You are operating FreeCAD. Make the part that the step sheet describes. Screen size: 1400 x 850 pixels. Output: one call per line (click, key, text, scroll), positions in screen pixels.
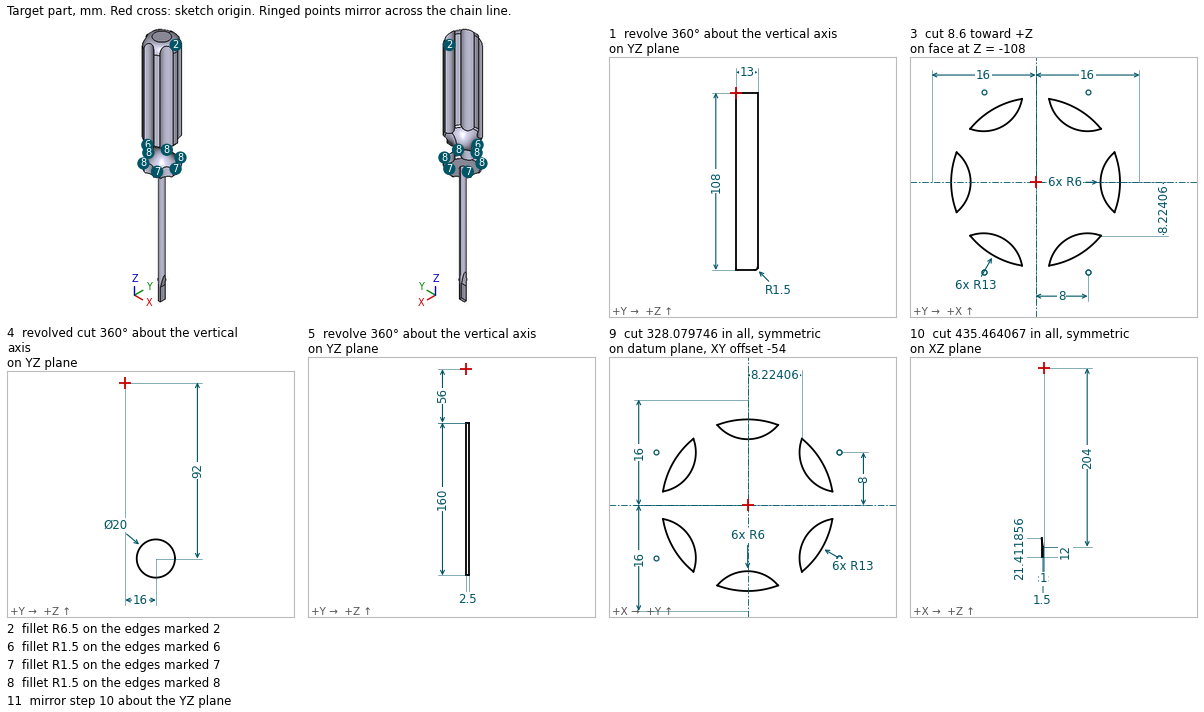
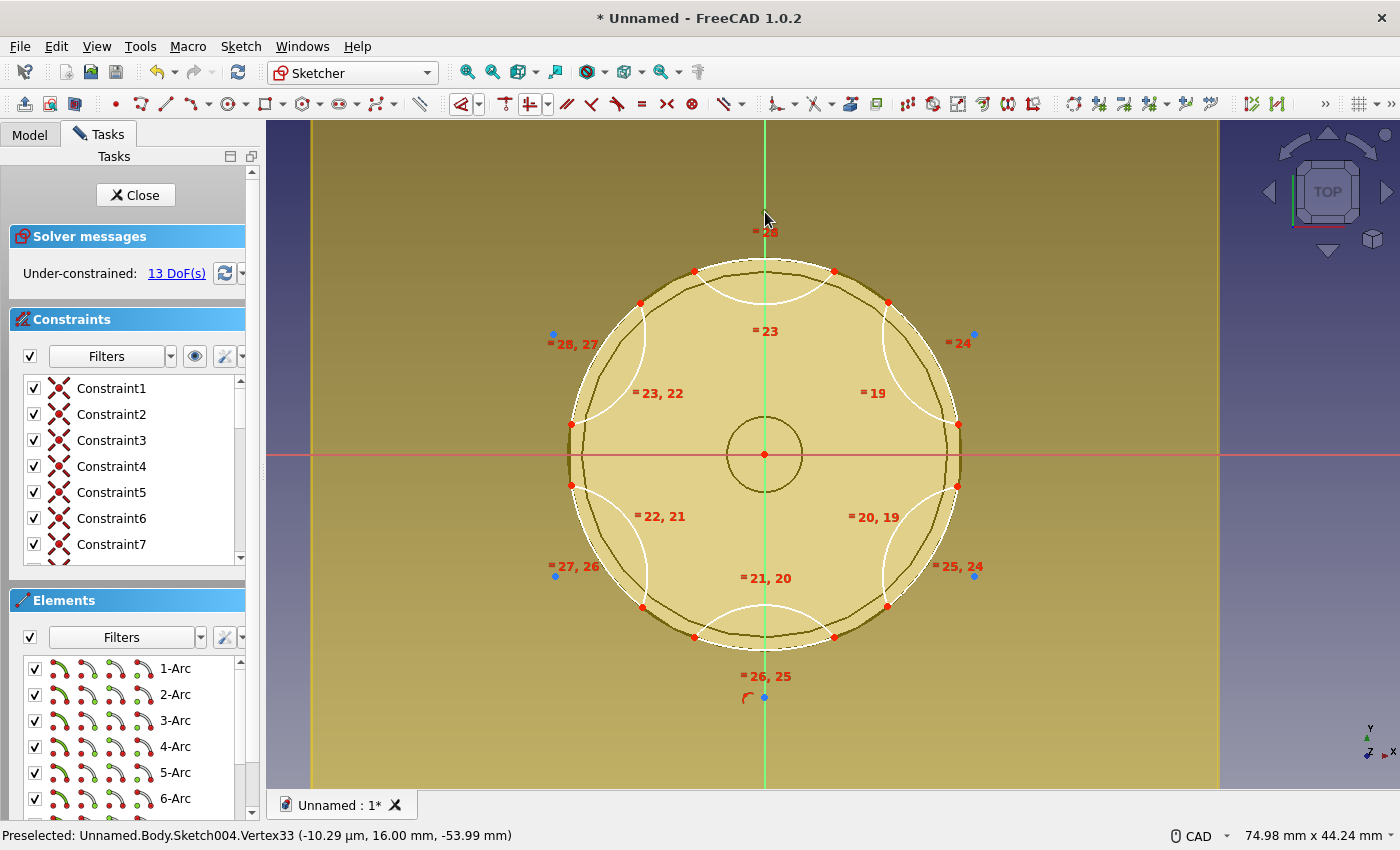
click(765, 717)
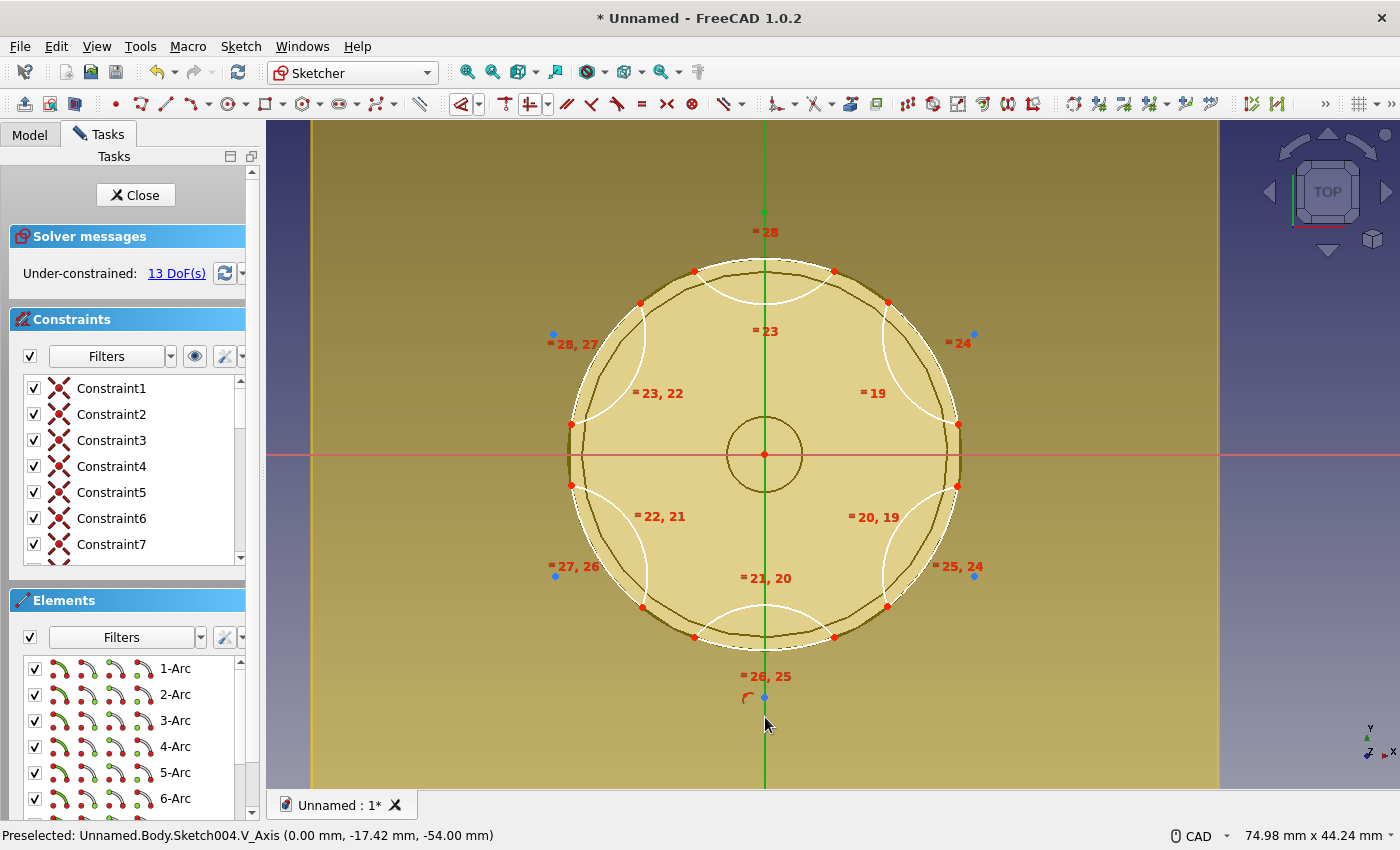
key(c)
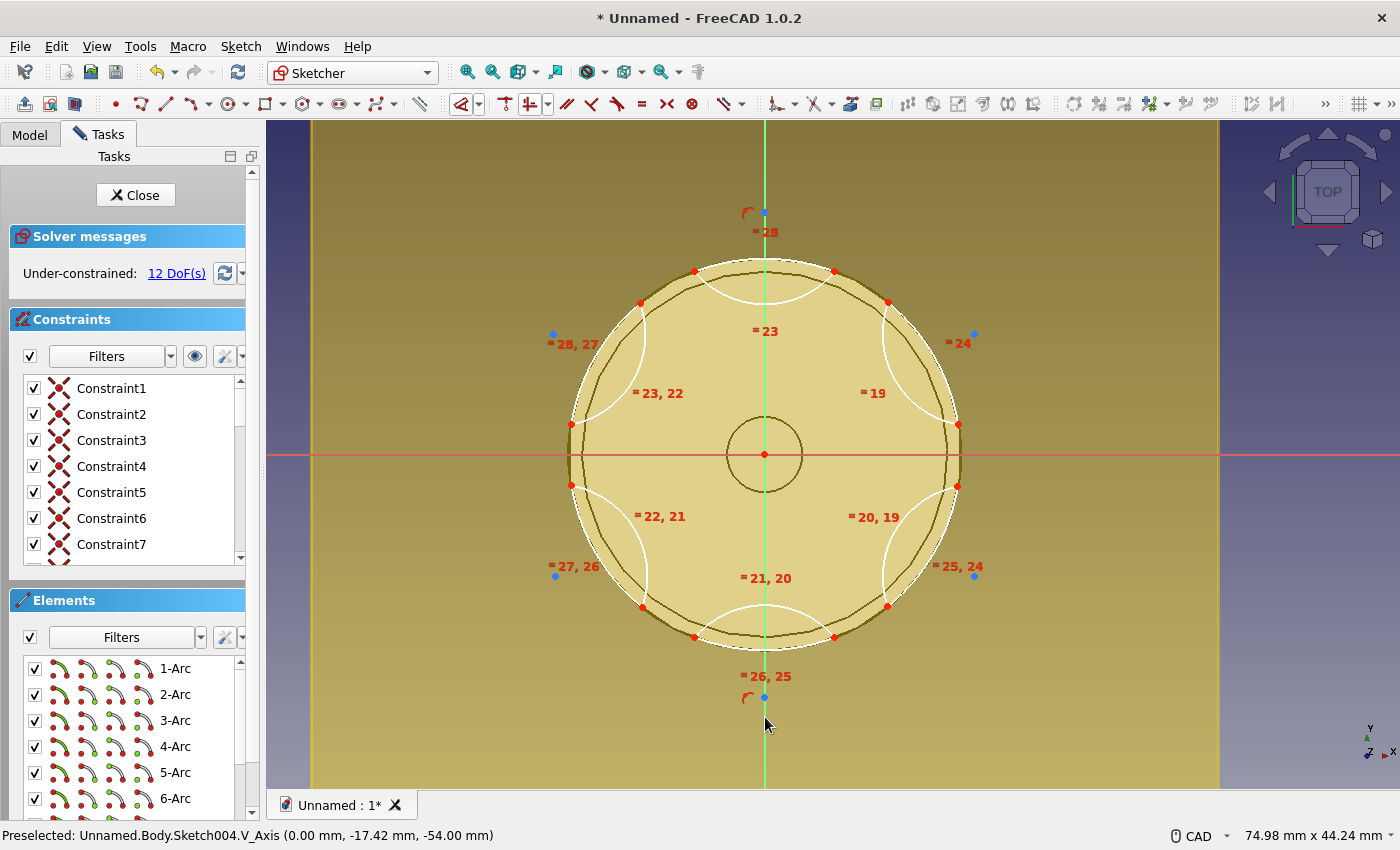
click(975, 334)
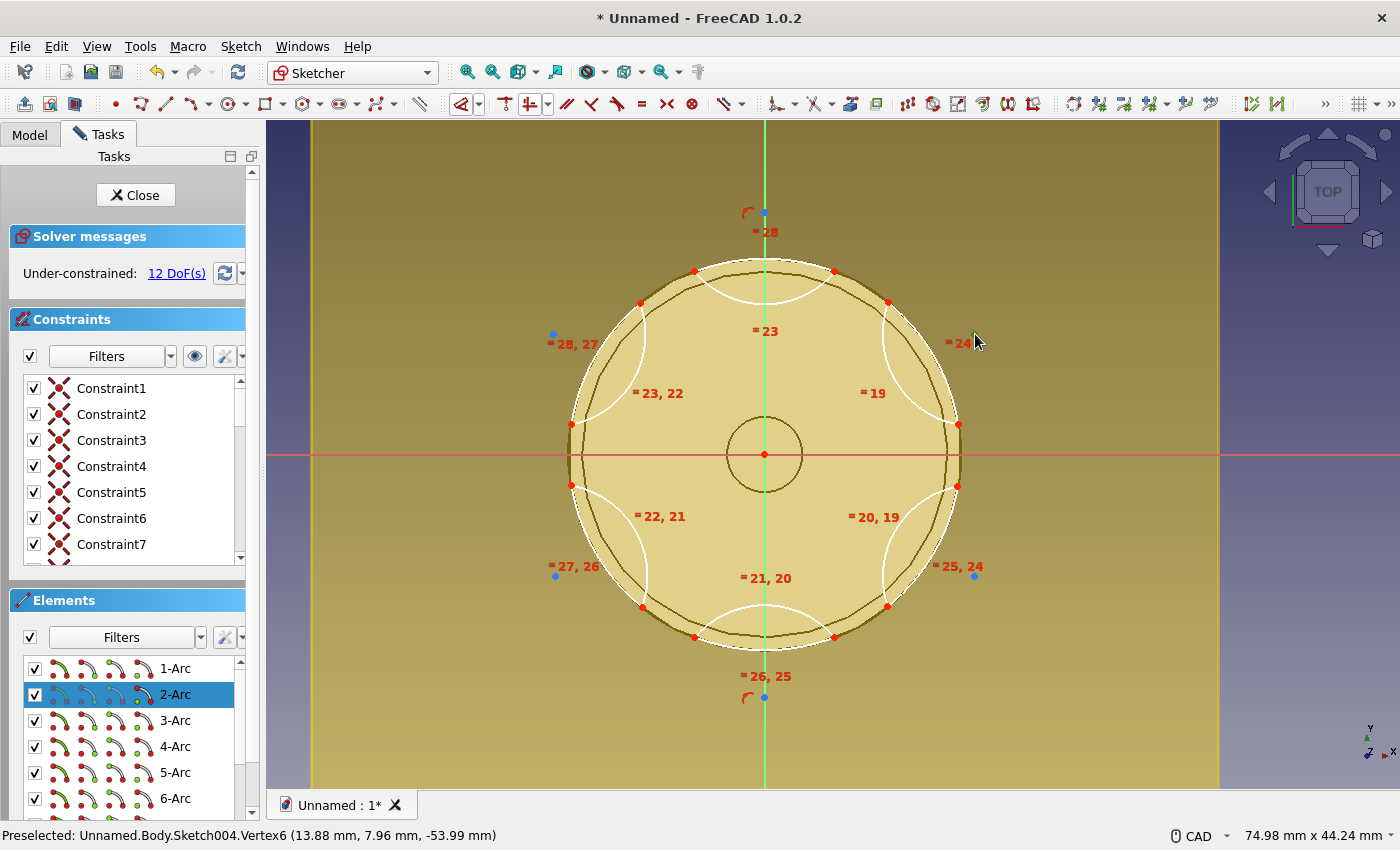
click(975, 577)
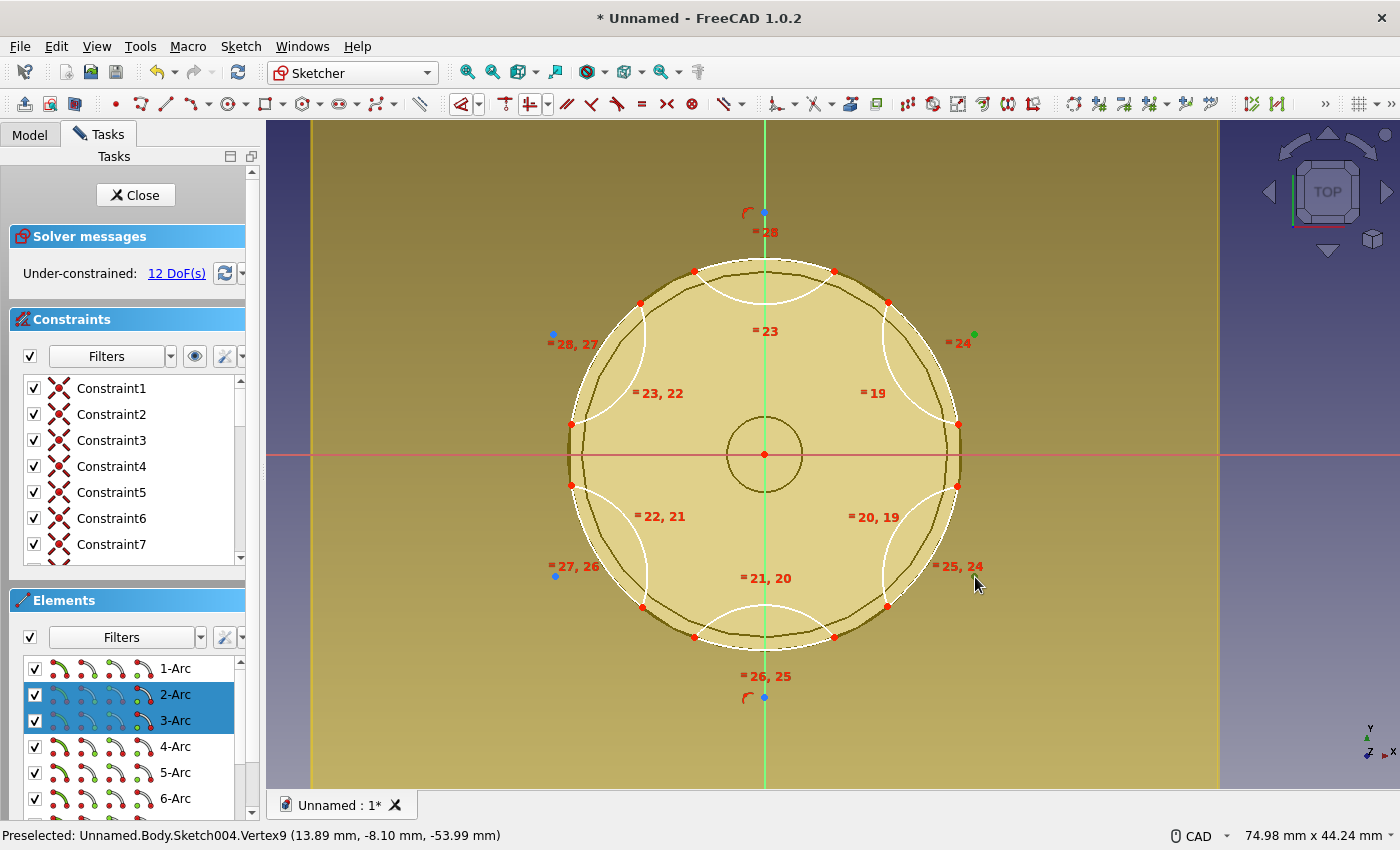
click(361, 455)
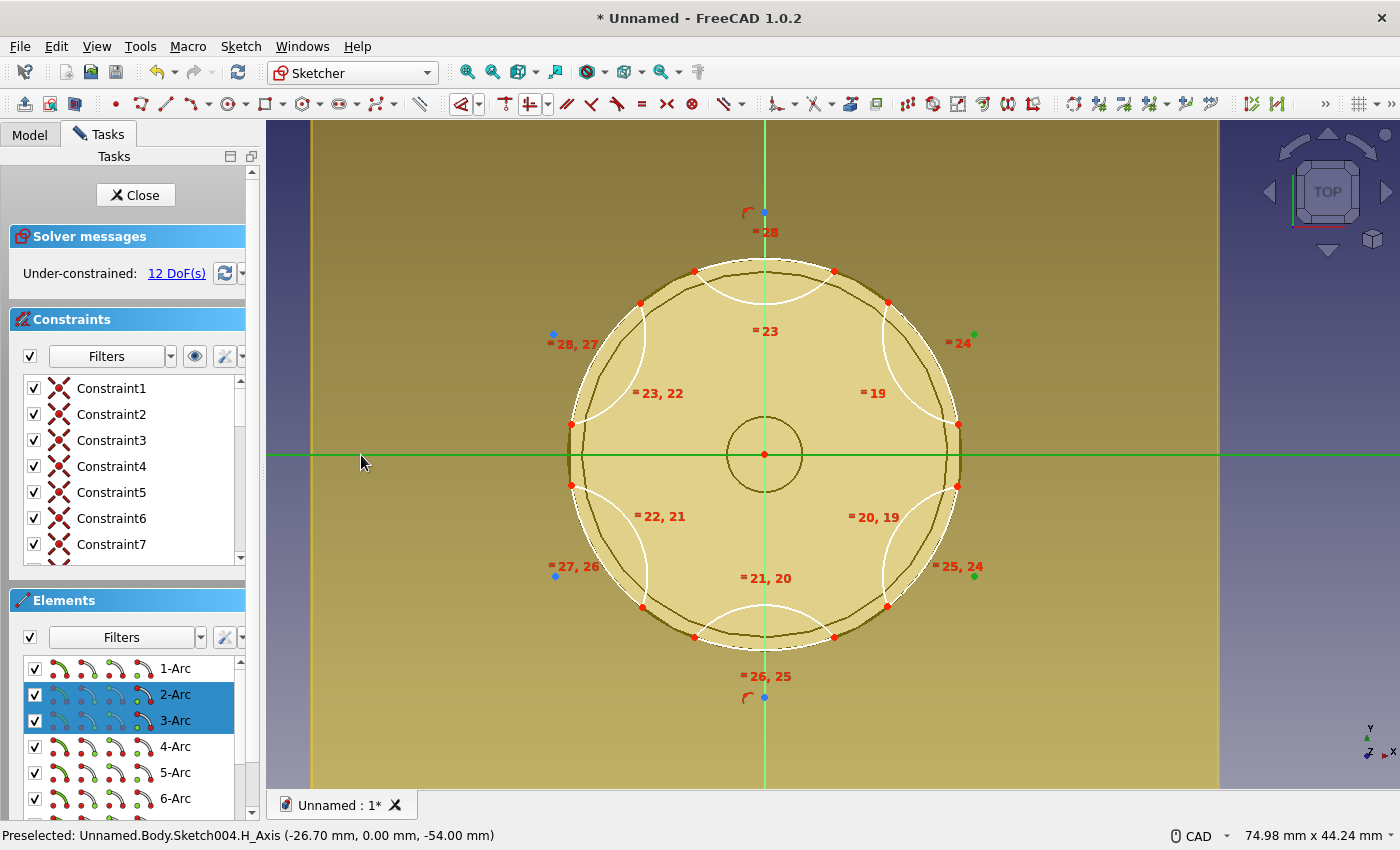
key(s)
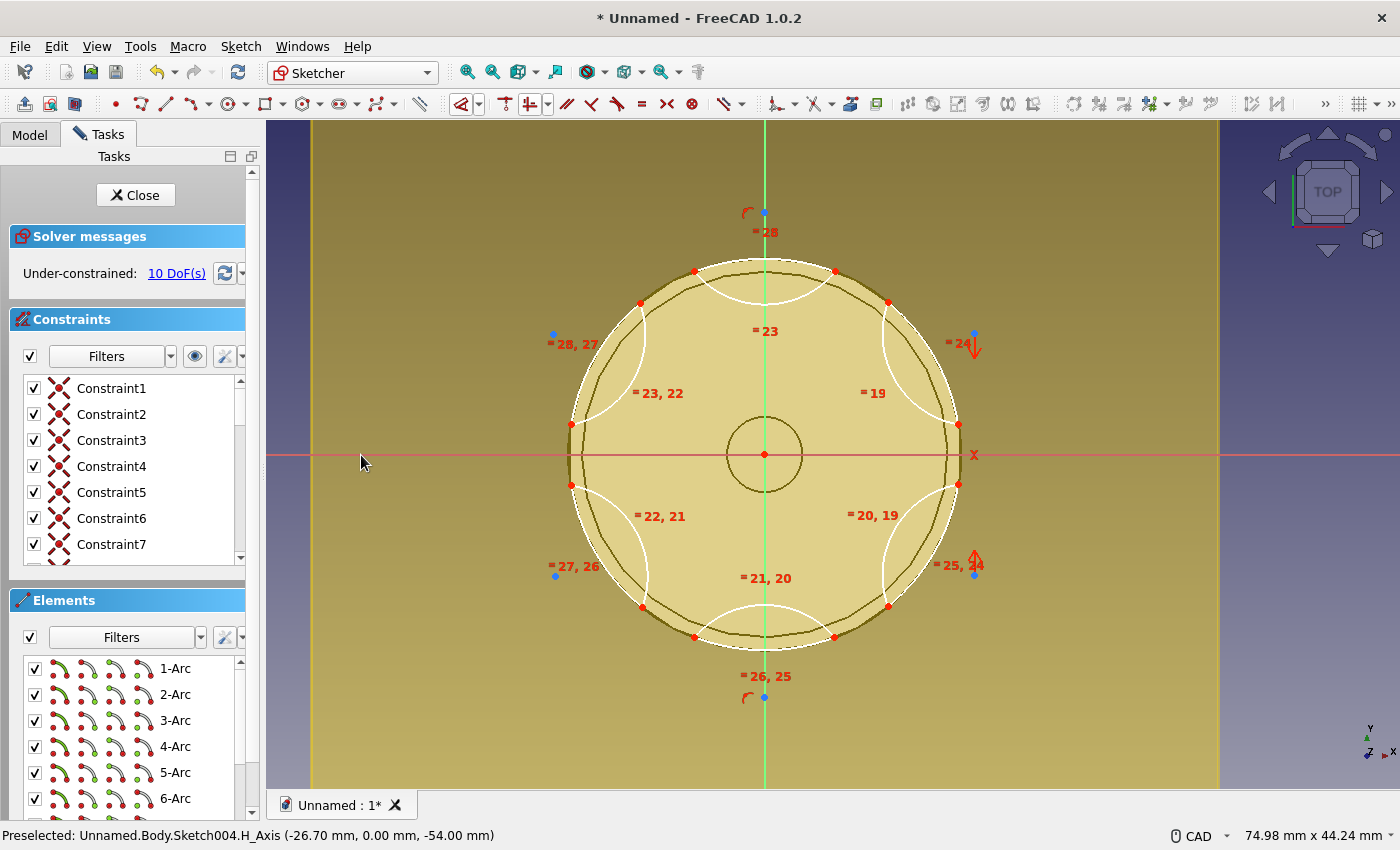
click(975, 575)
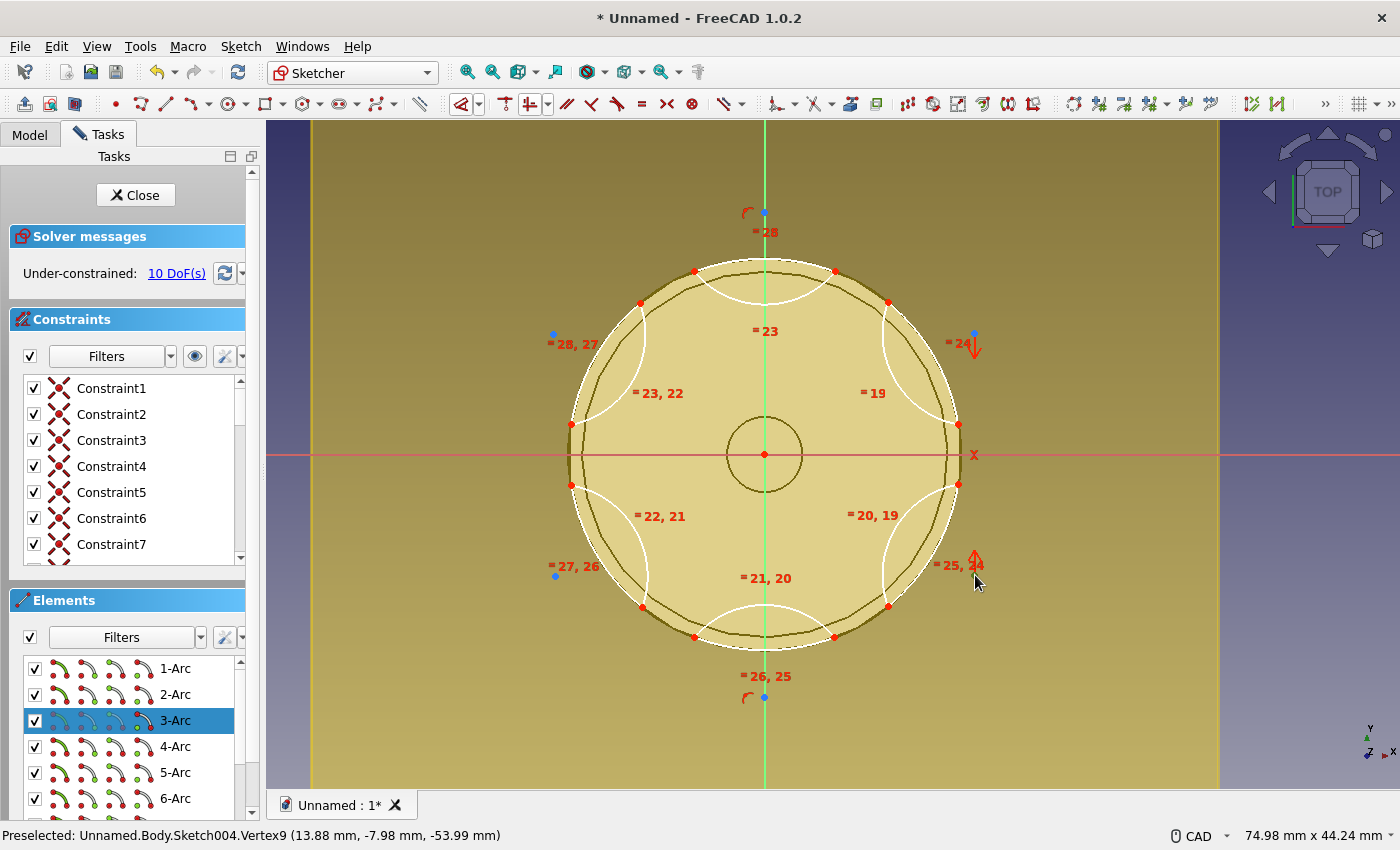
click(556, 576)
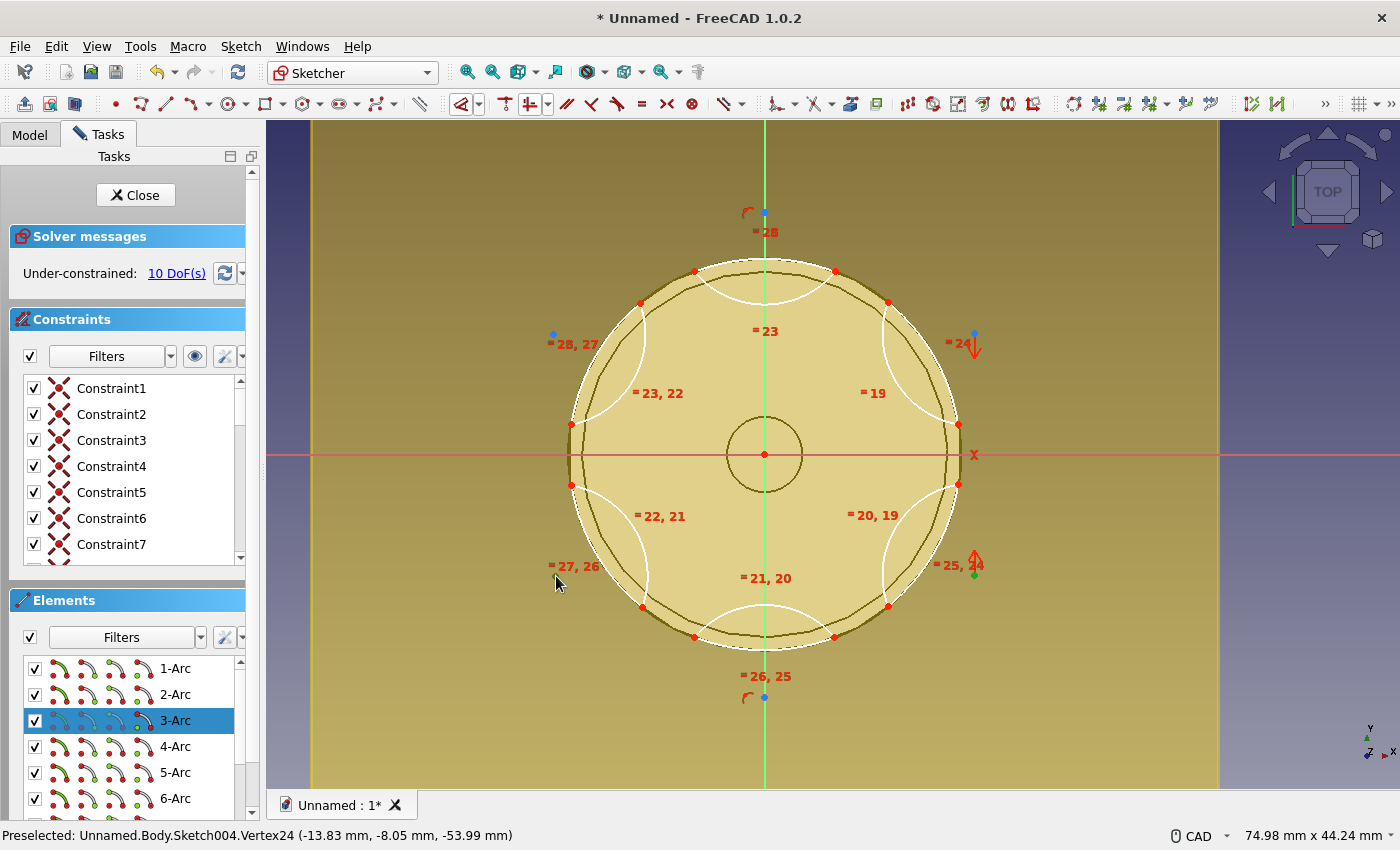
click(765, 717)